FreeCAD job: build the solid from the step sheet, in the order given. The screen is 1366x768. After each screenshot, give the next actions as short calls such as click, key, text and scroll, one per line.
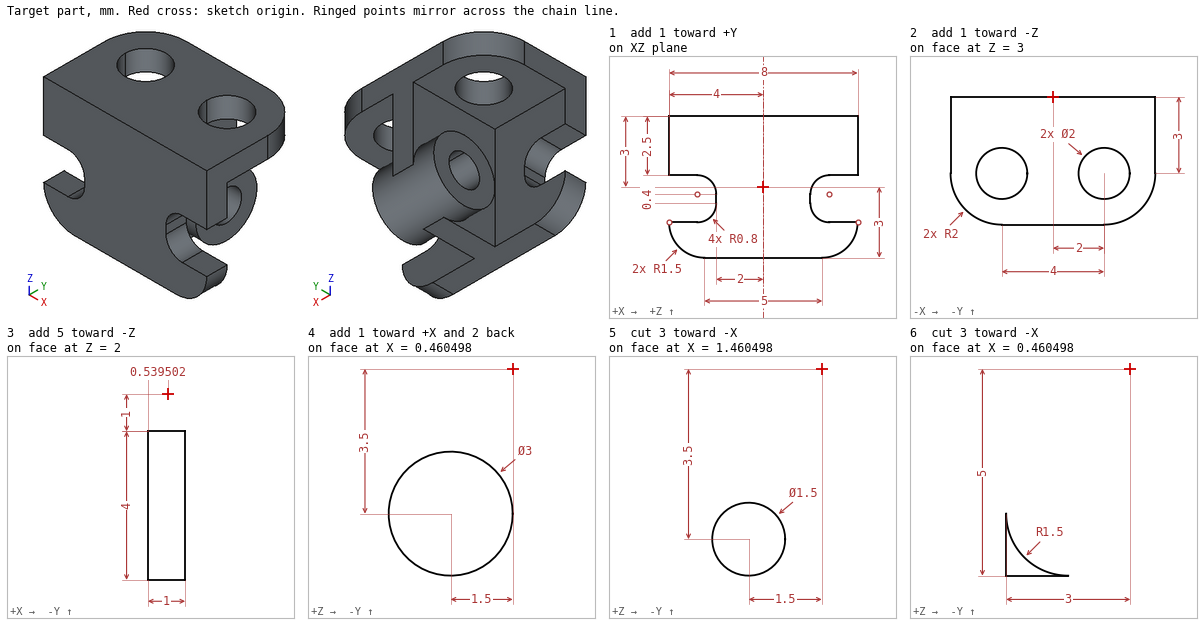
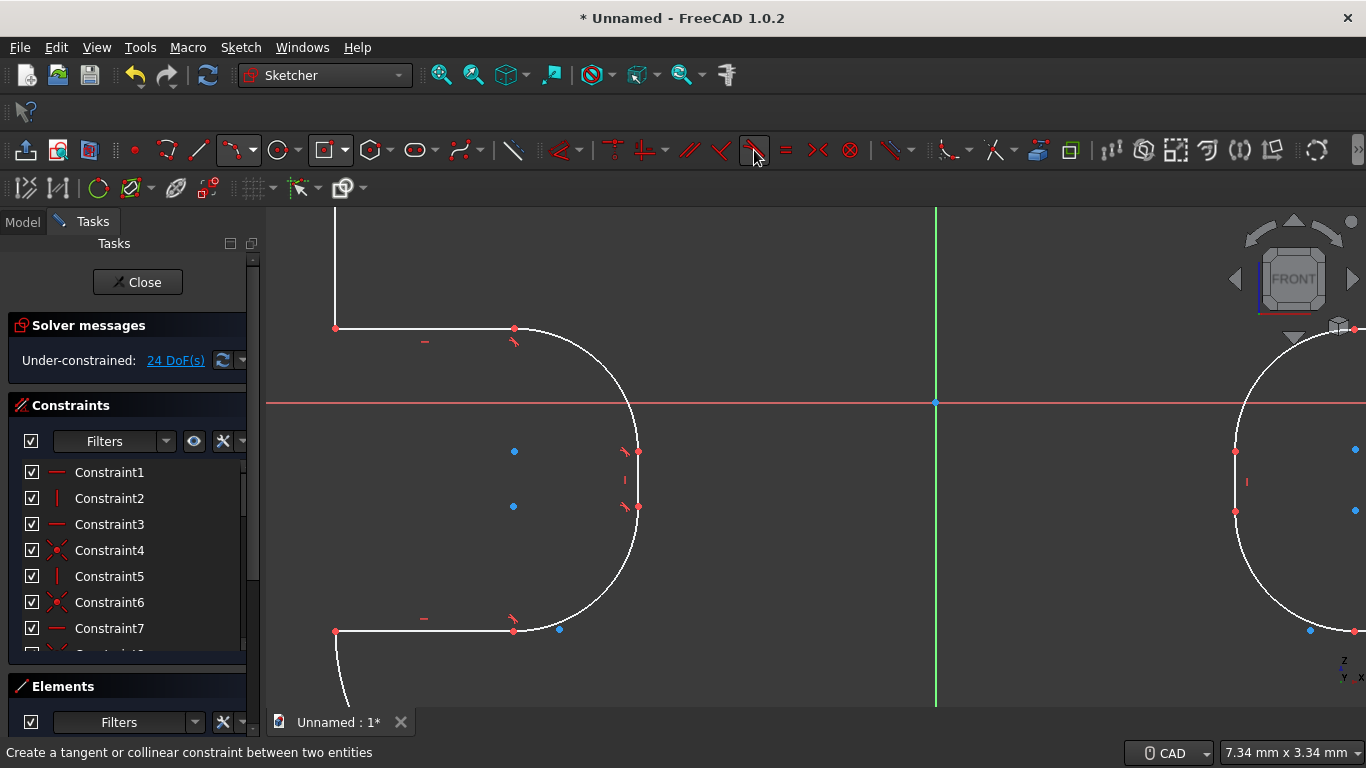
scroll(638, 489, down, 5)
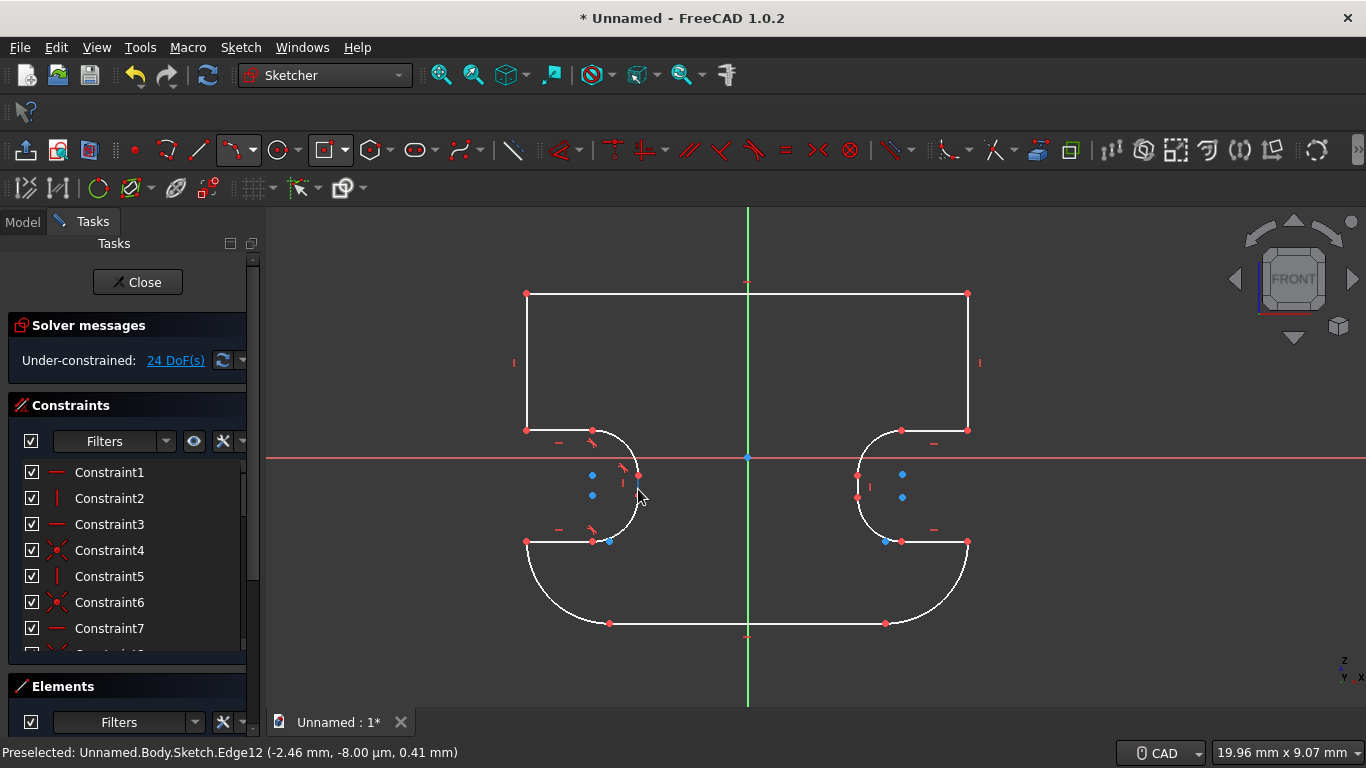
click(948, 431)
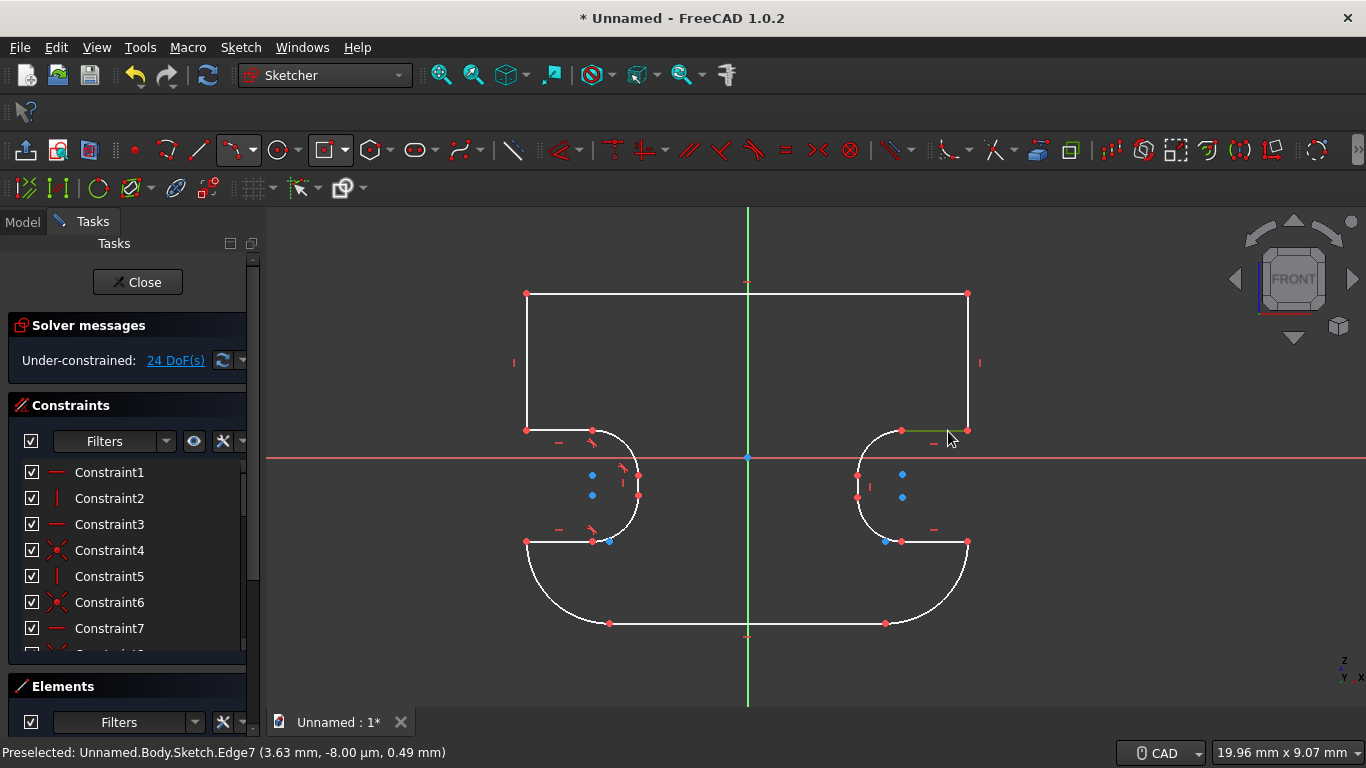
click(882, 436)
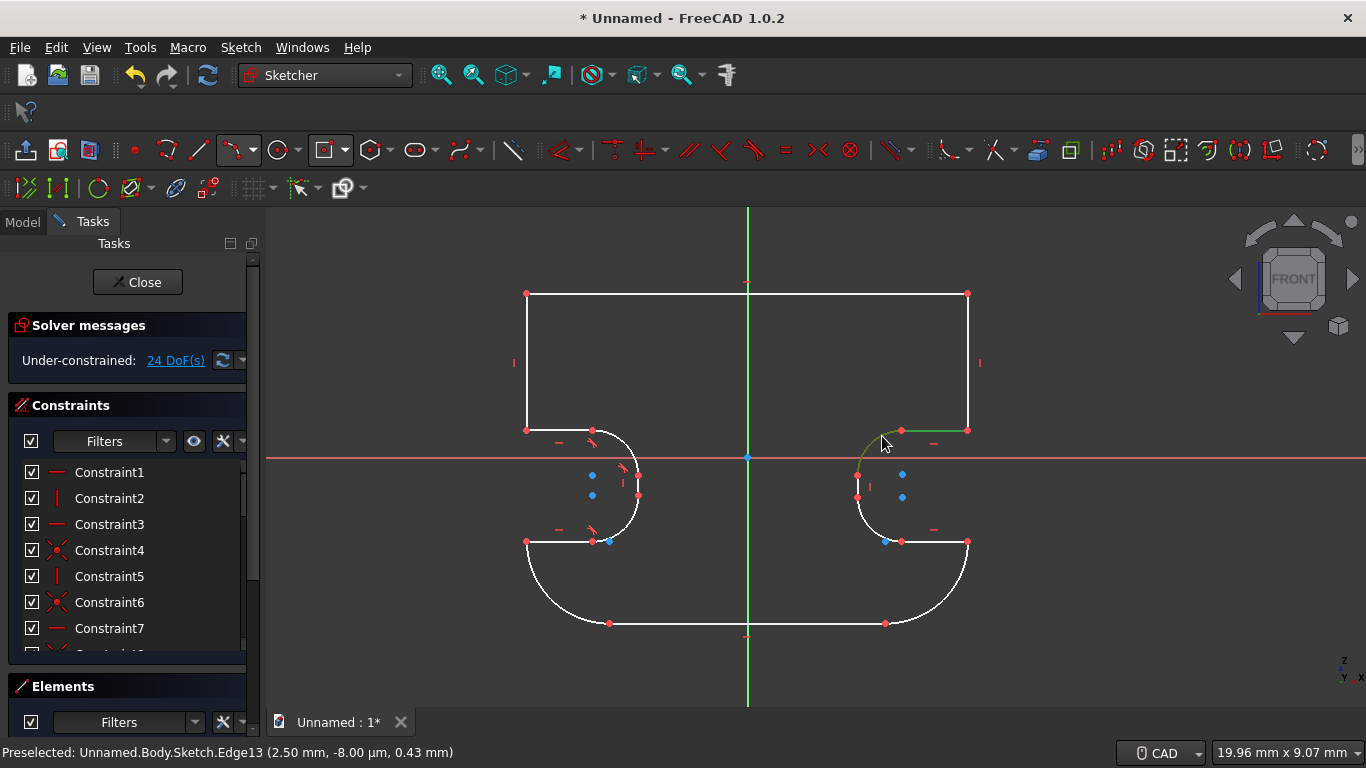
click(754, 150)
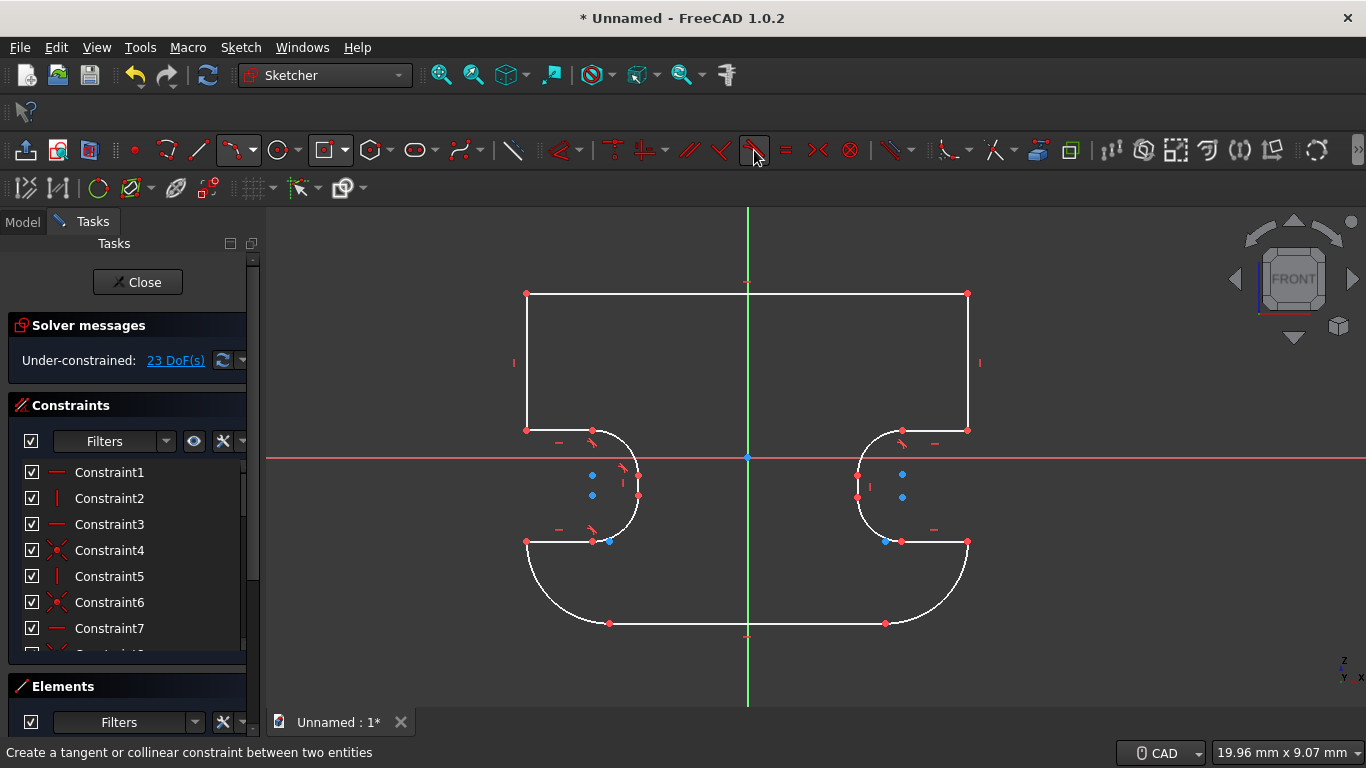
scroll(858, 487, up, 2)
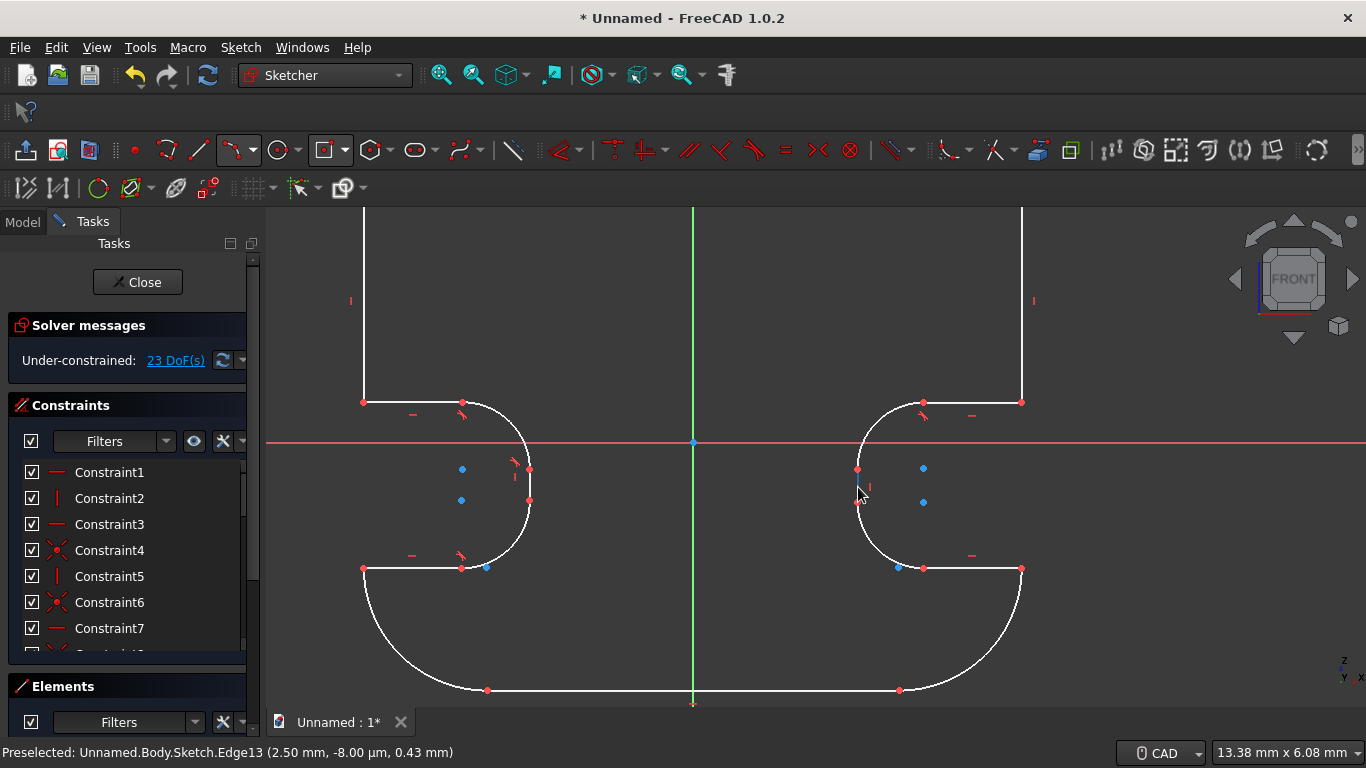
click(858, 486)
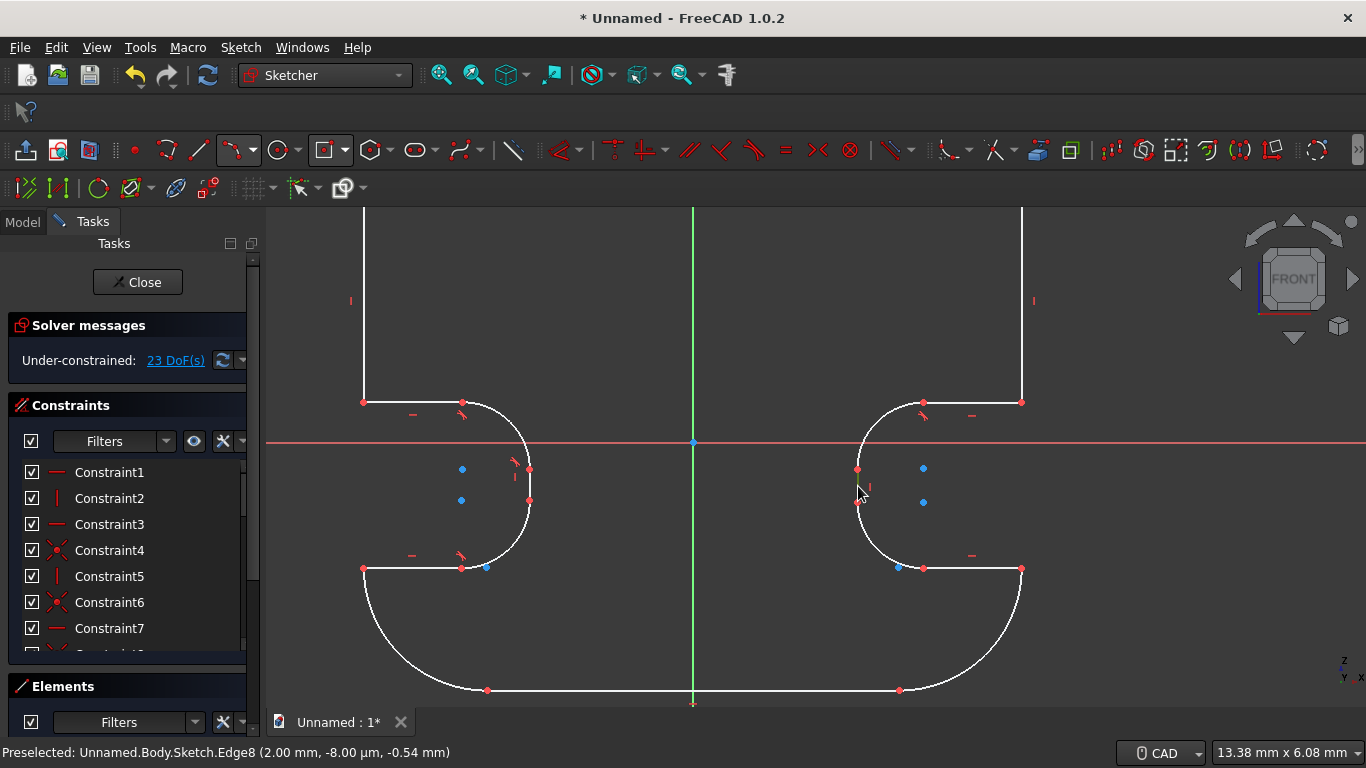
click(893, 410)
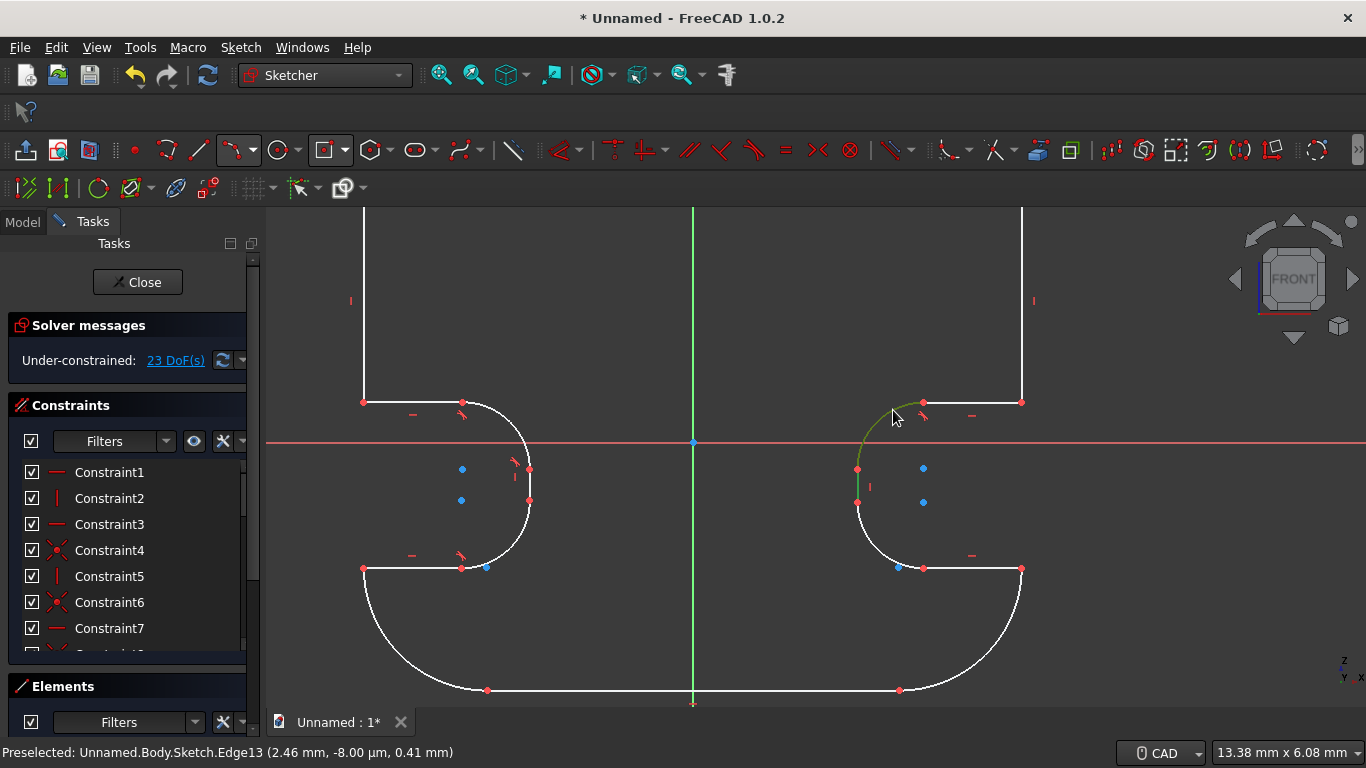
click(754, 150)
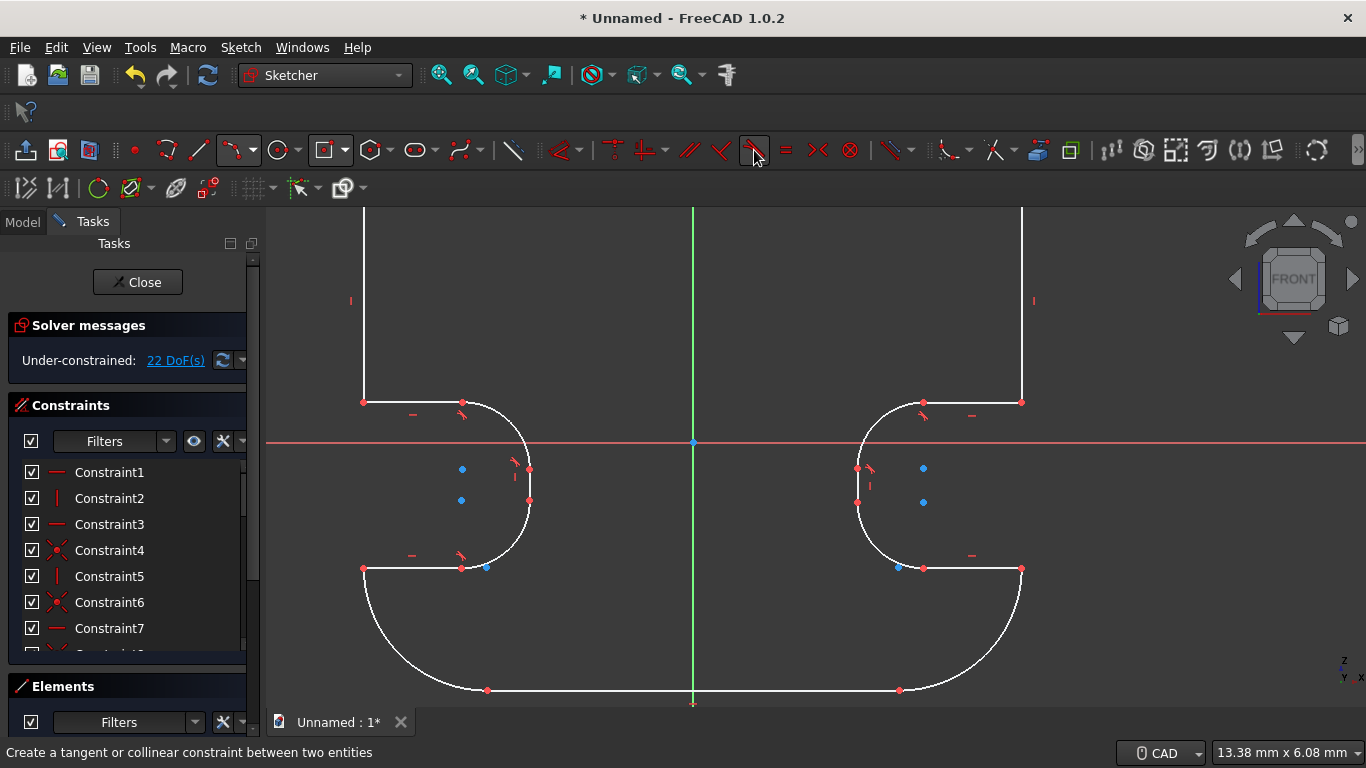
scroll(858, 479, up, 2)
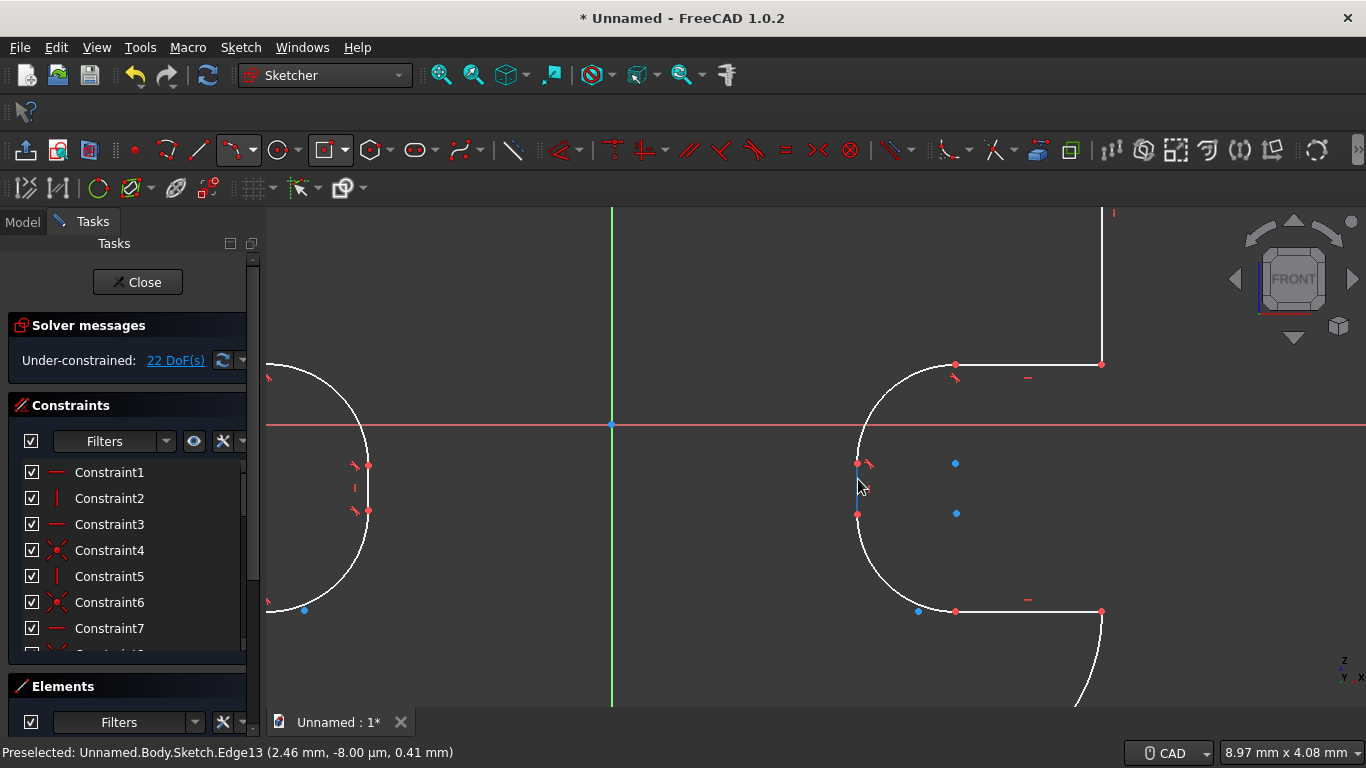
click(857, 479)